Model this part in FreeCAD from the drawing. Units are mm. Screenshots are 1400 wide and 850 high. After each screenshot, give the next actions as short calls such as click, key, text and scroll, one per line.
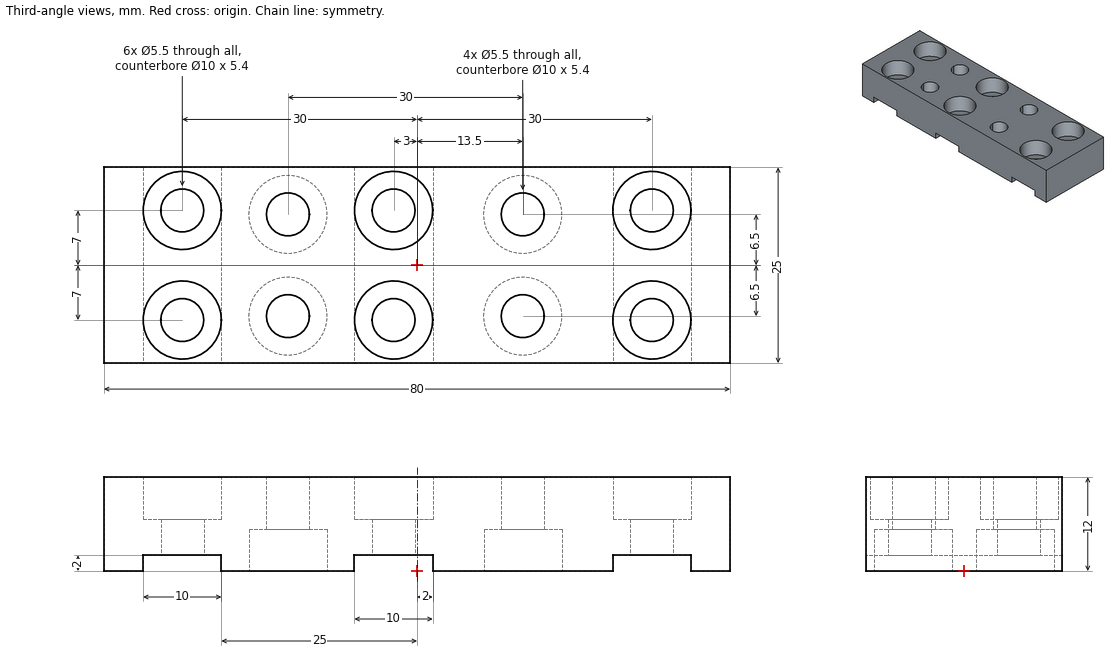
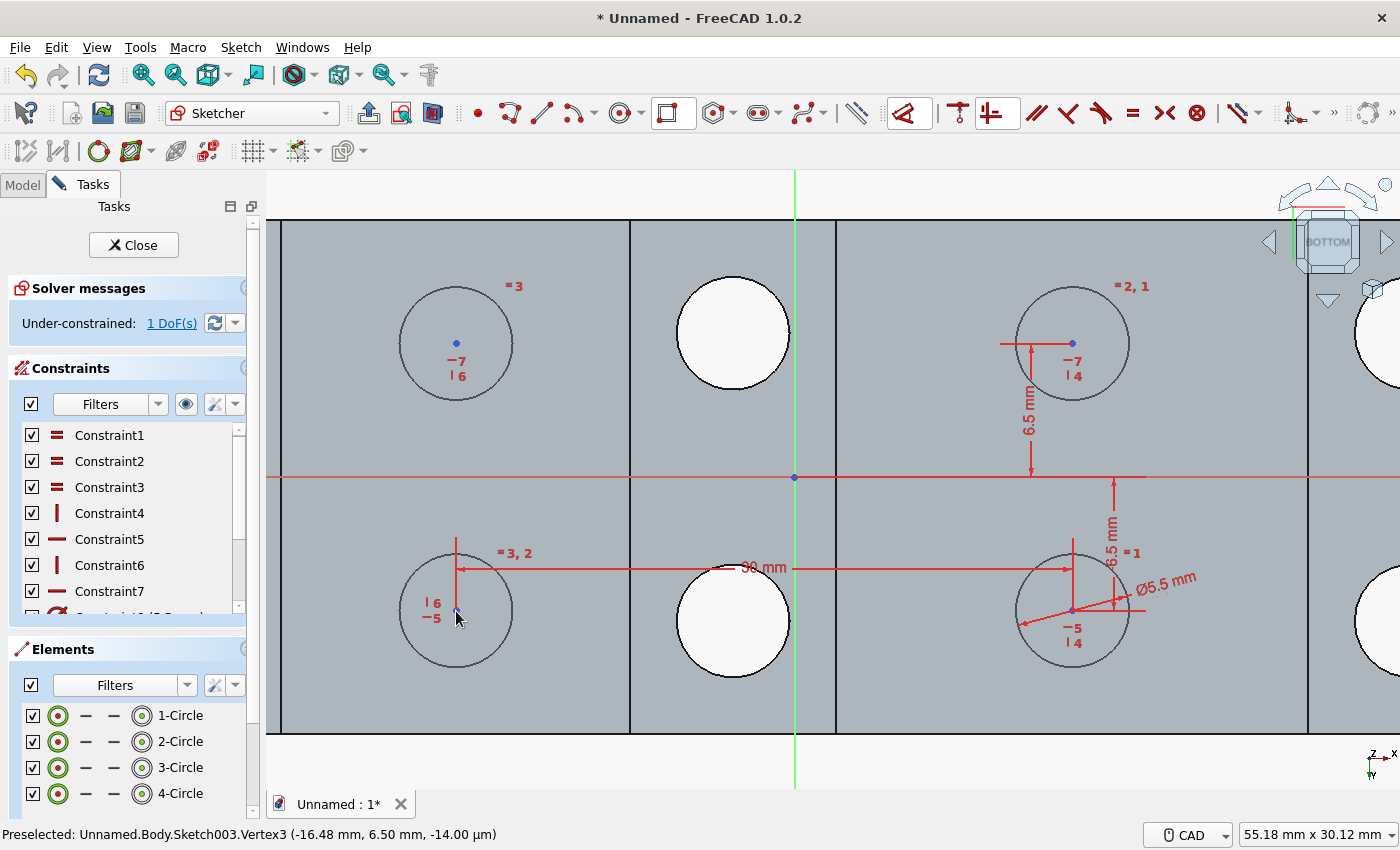
click(1073, 611)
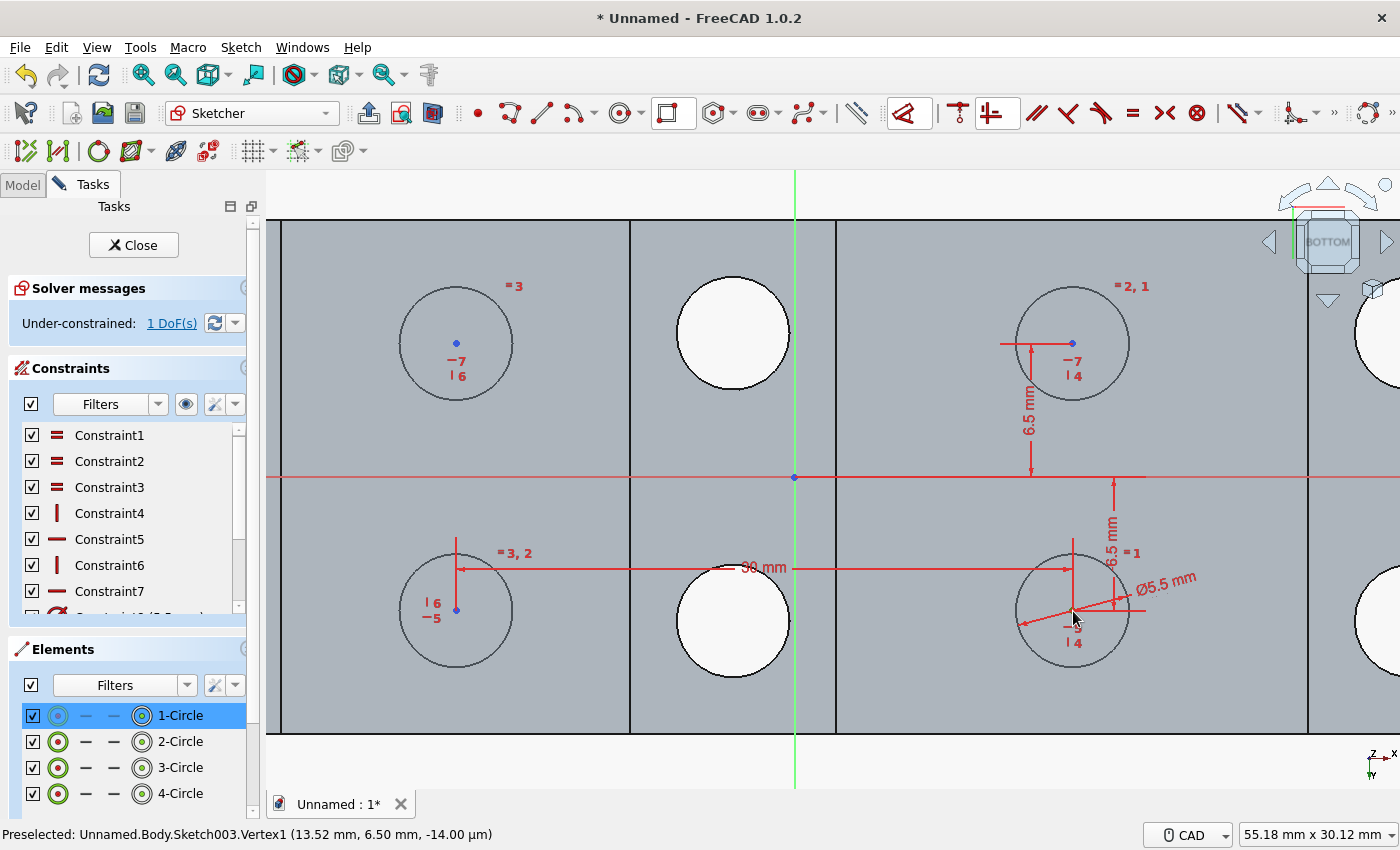
key(l)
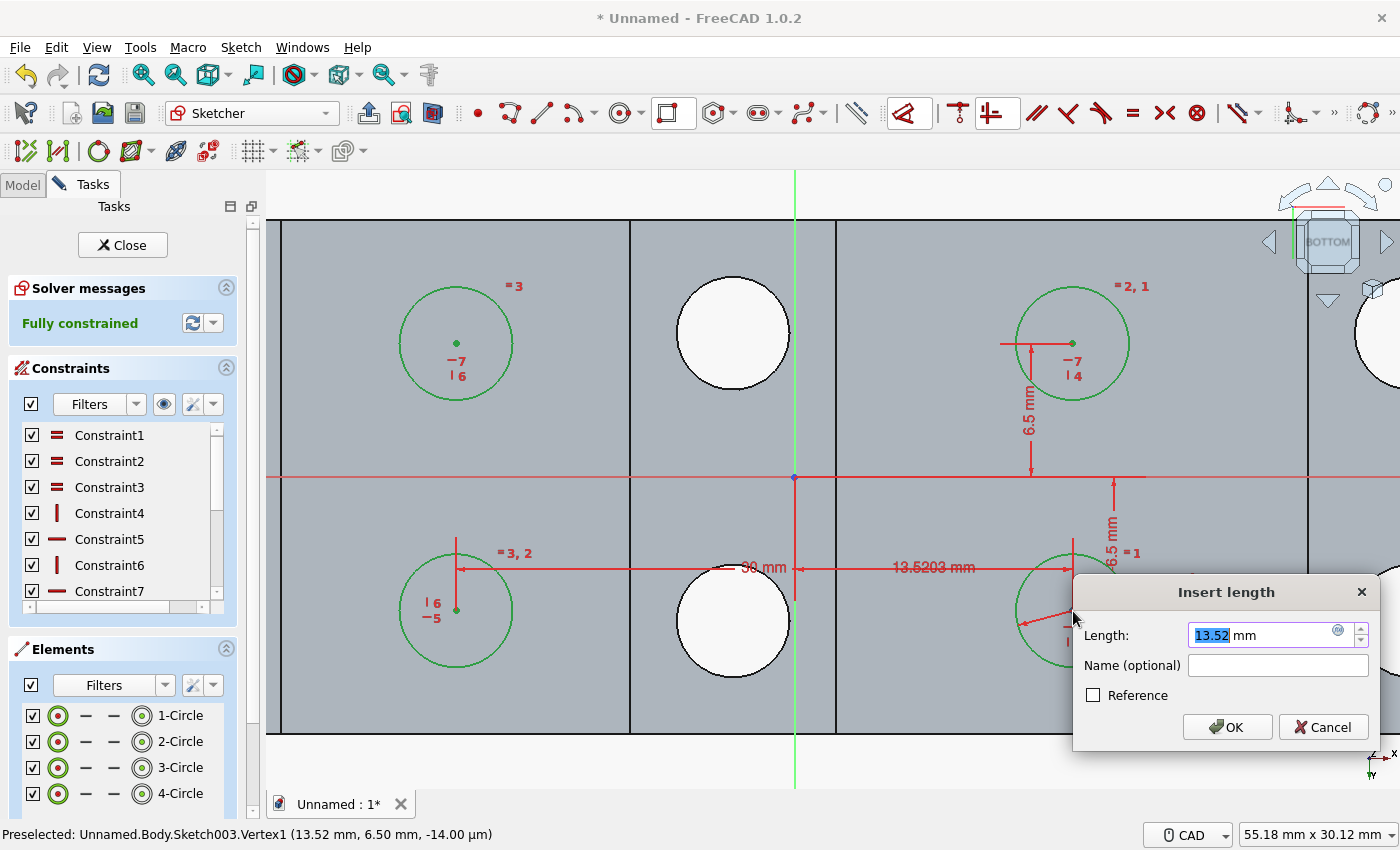
text(13.5)
key(Return)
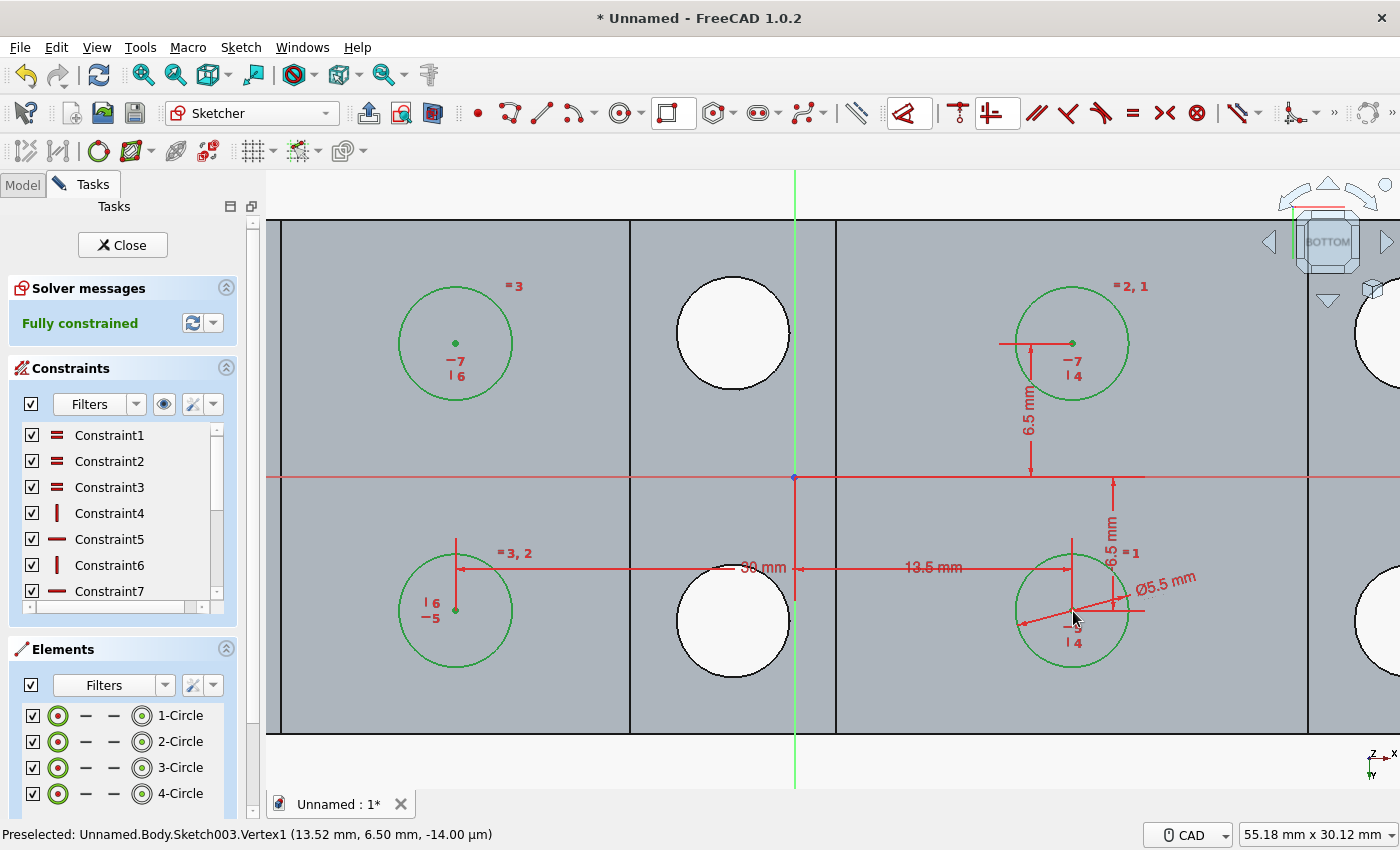
click(123, 245)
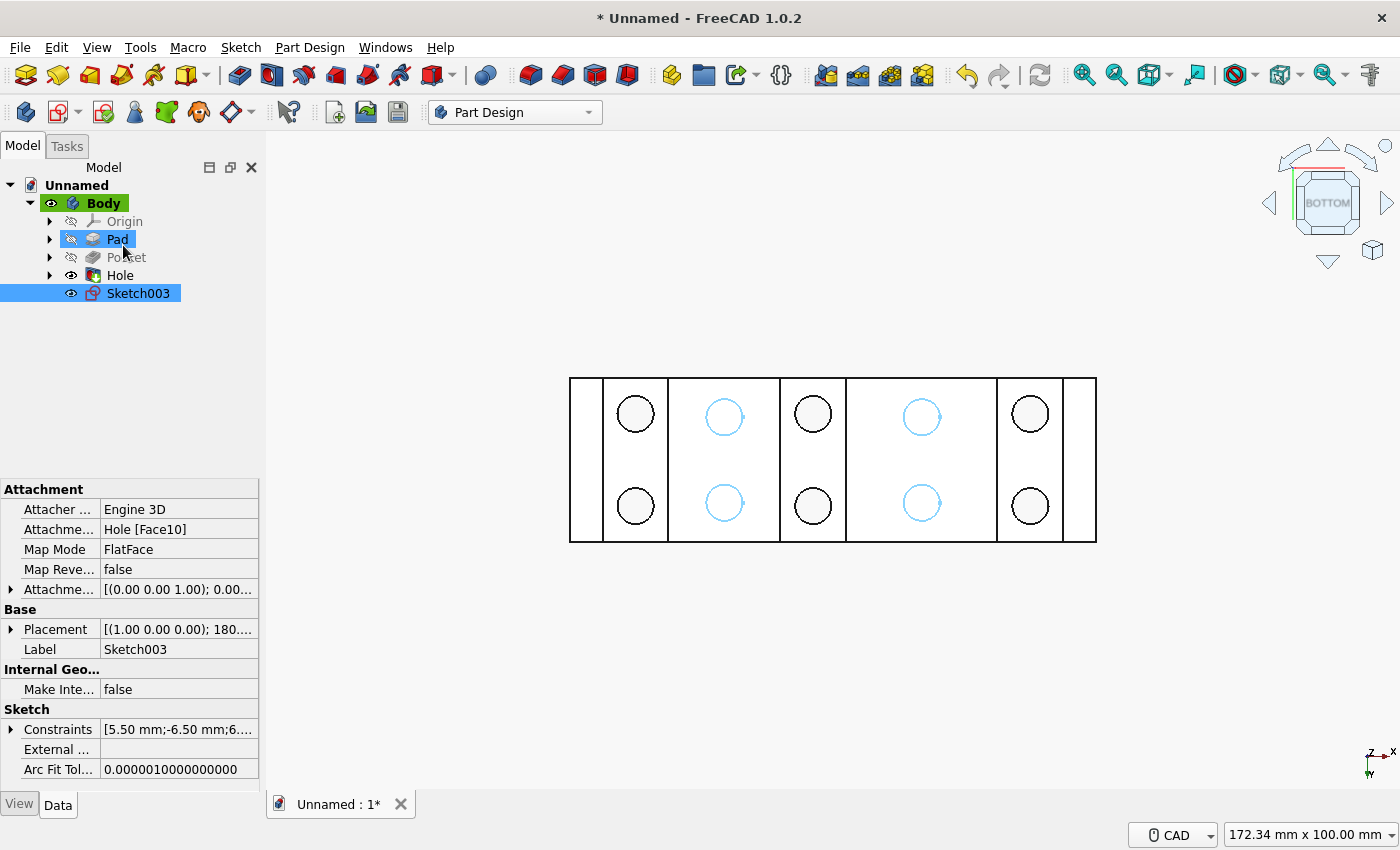
click(272, 76)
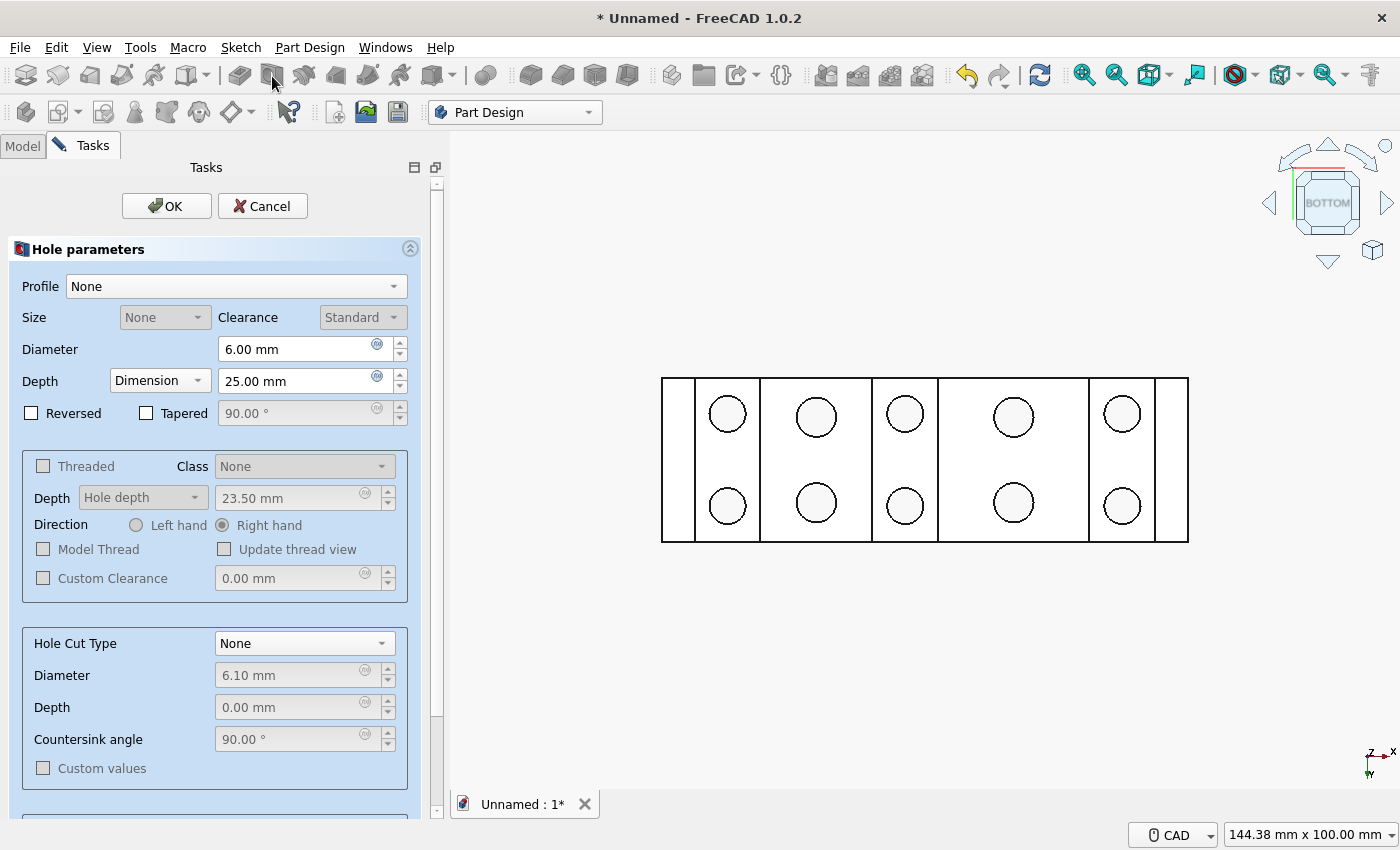
triple_click(305, 349)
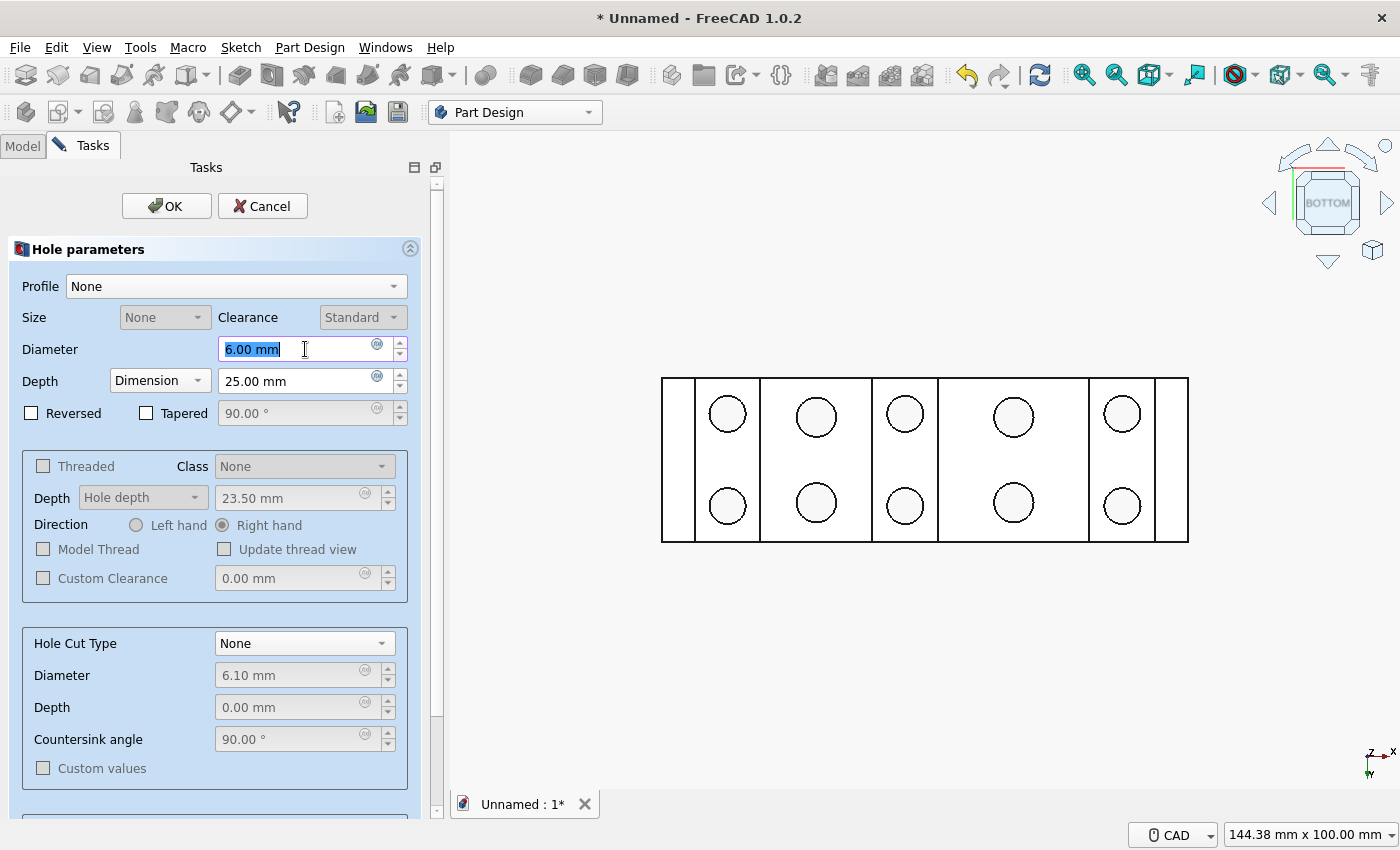
text(5.5)
key(Tab)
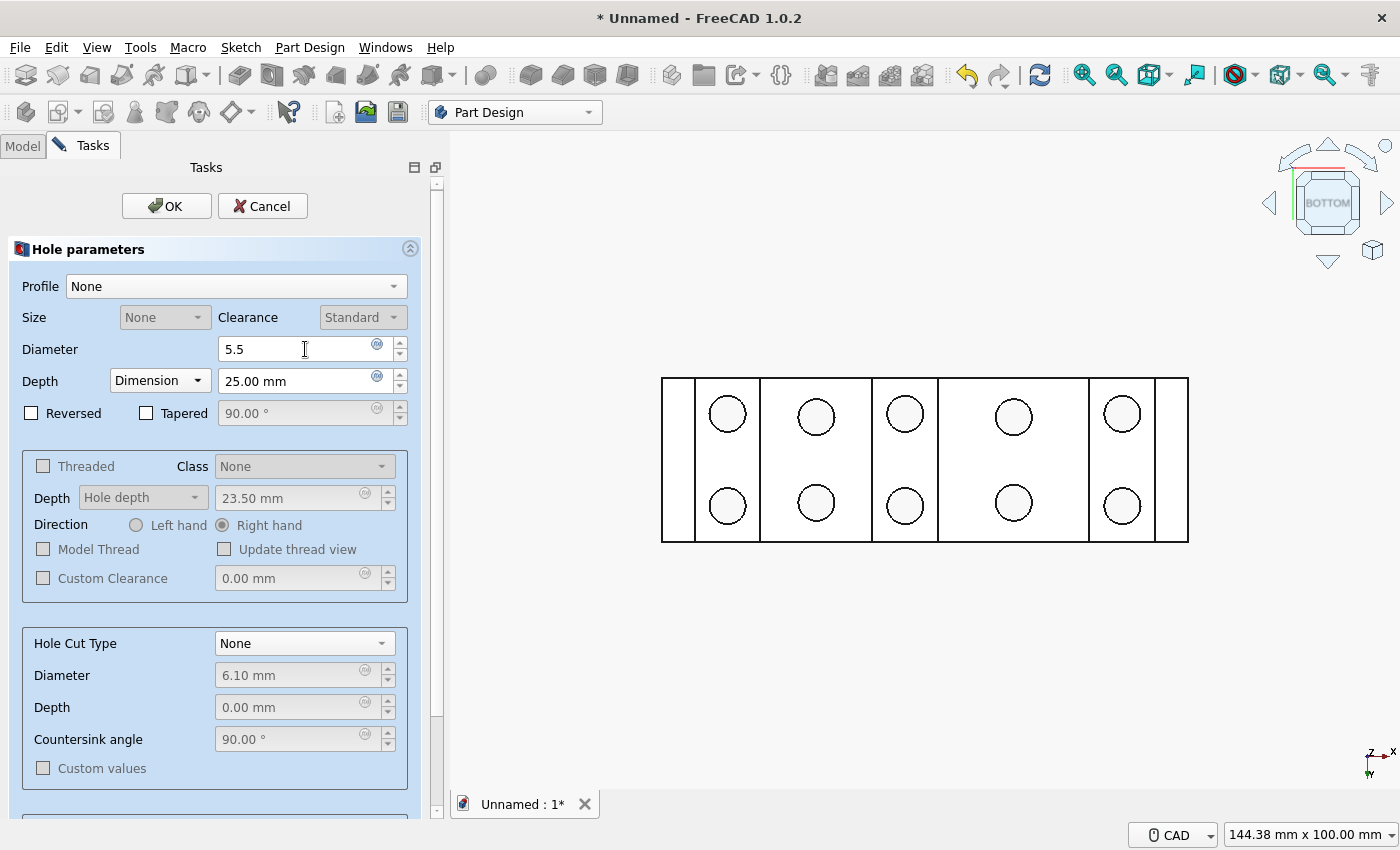
click(161, 380)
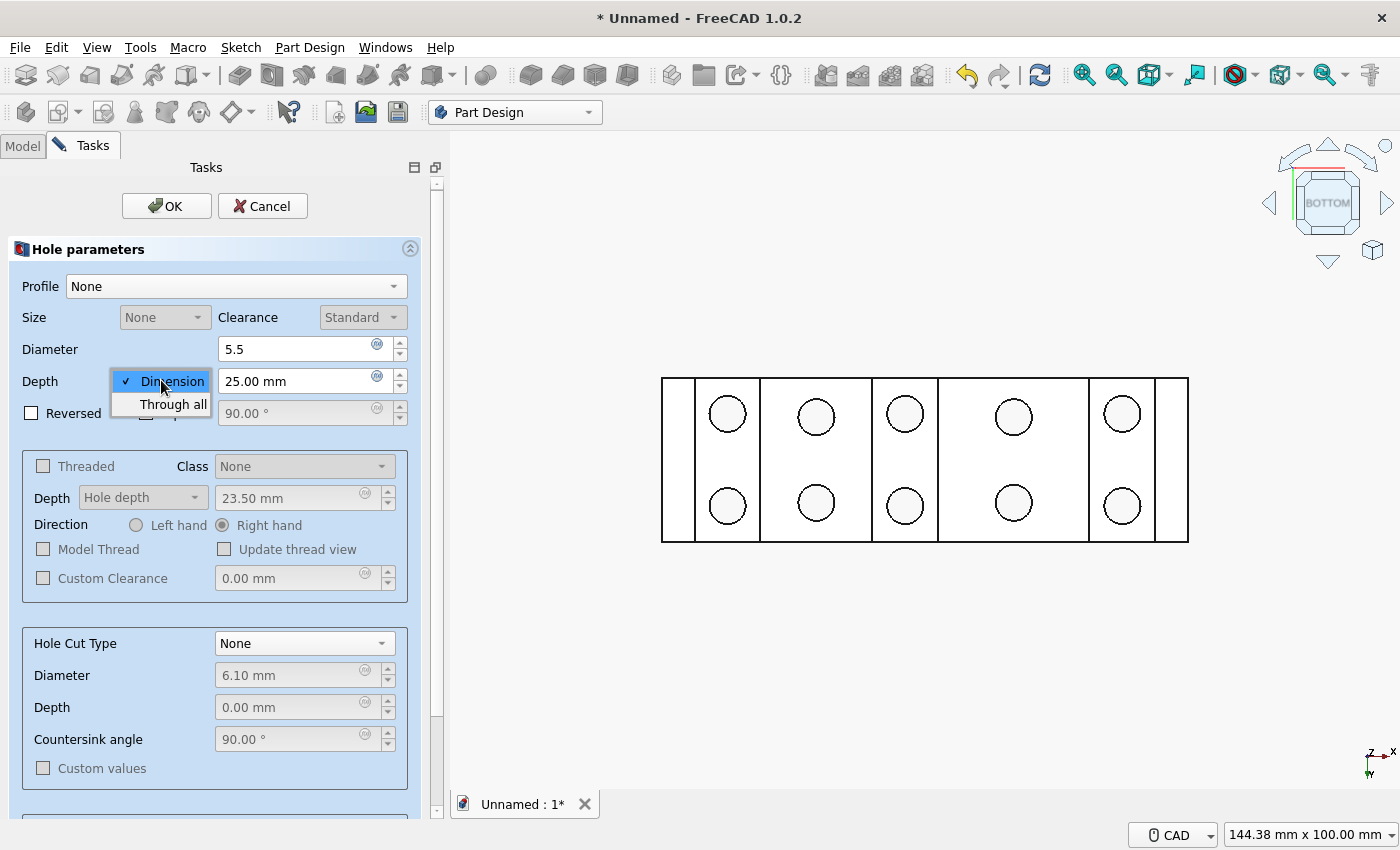
click(160, 404)